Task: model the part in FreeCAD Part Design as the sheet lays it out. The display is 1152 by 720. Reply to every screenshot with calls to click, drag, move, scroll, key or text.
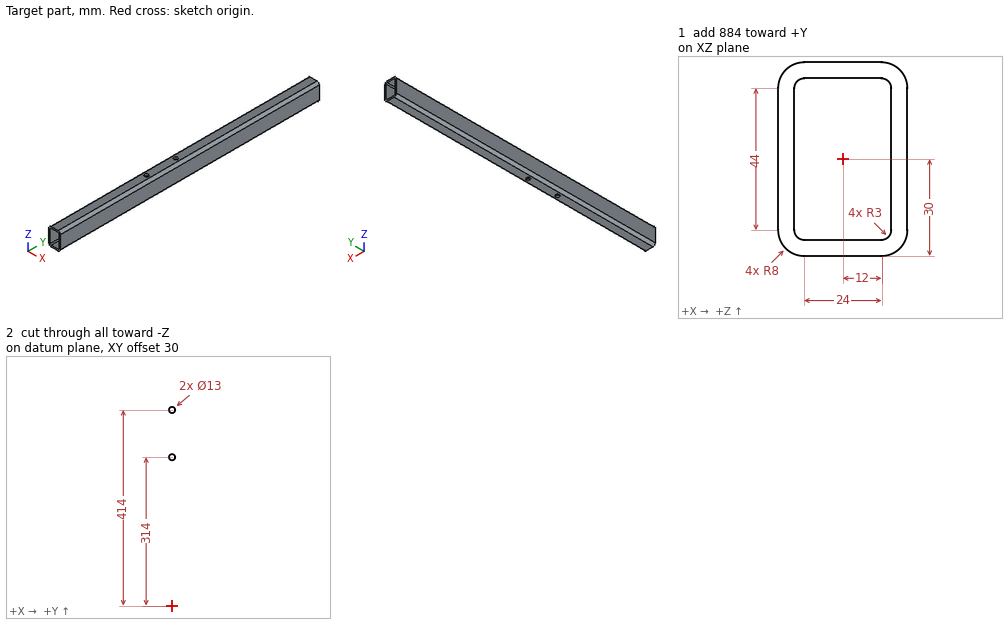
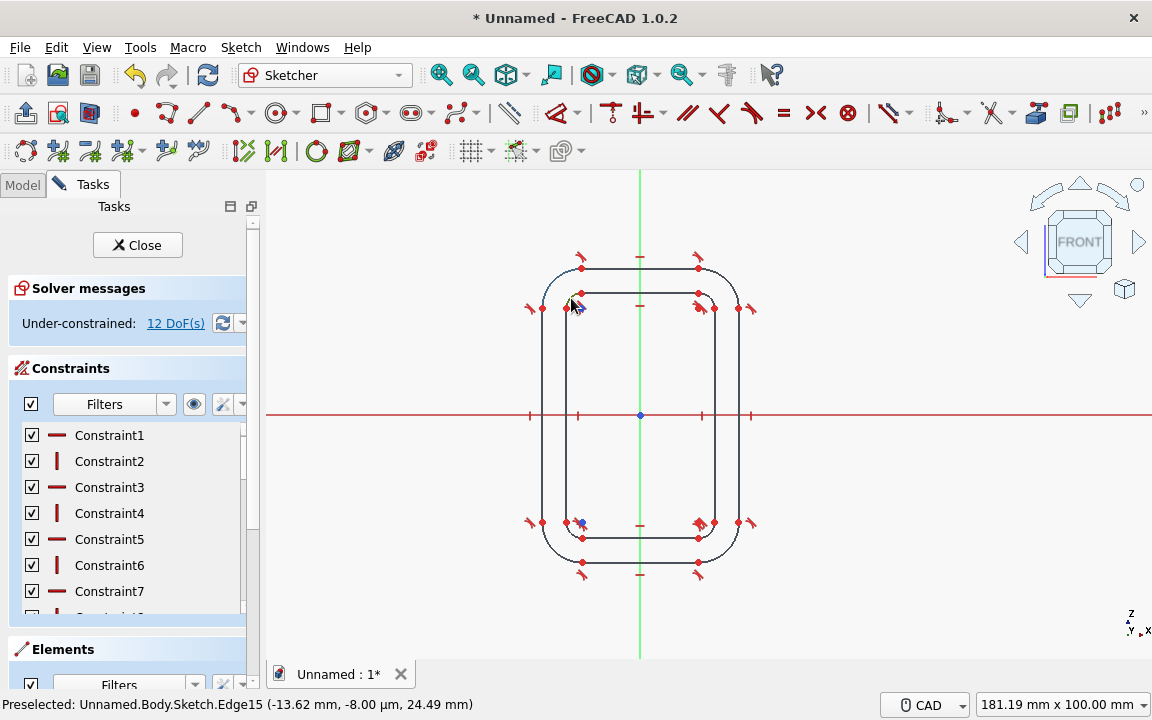
click(612, 114)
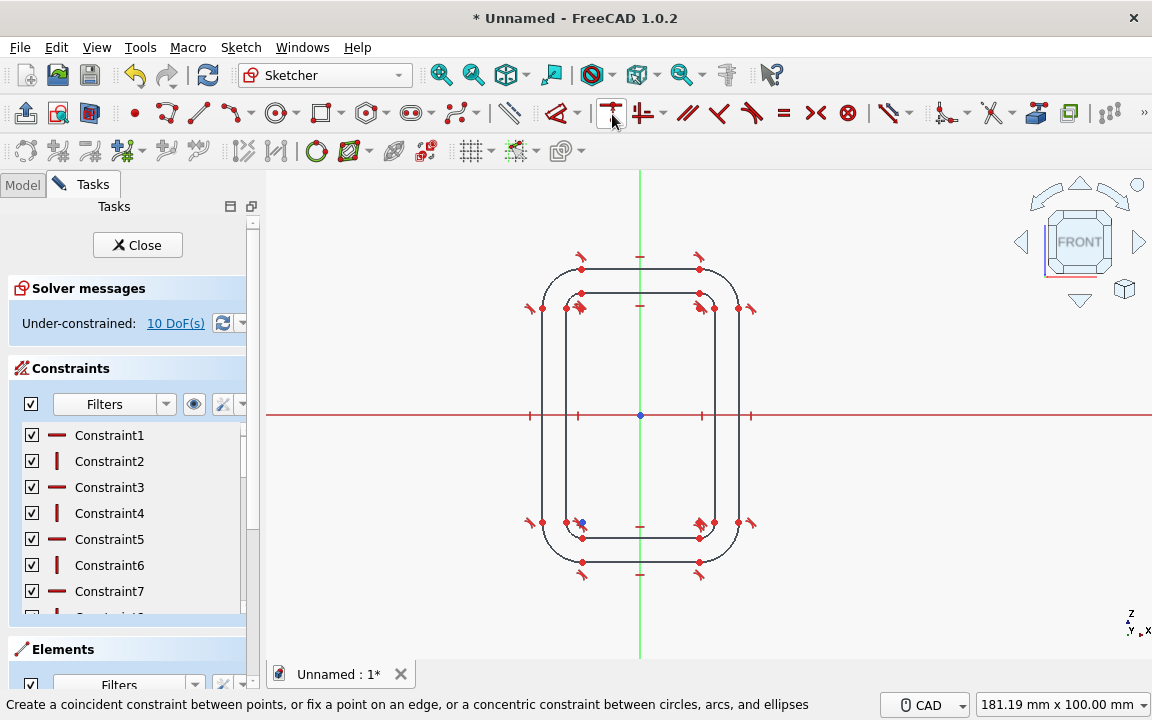
click(547, 541)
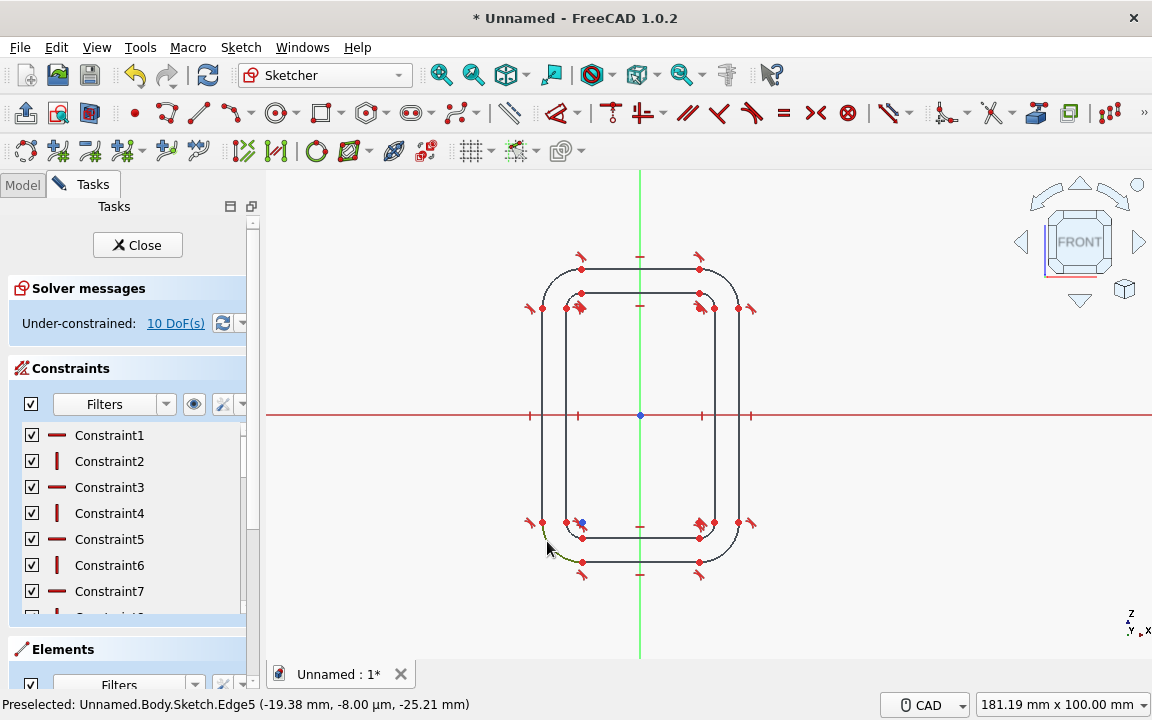
click(564, 273)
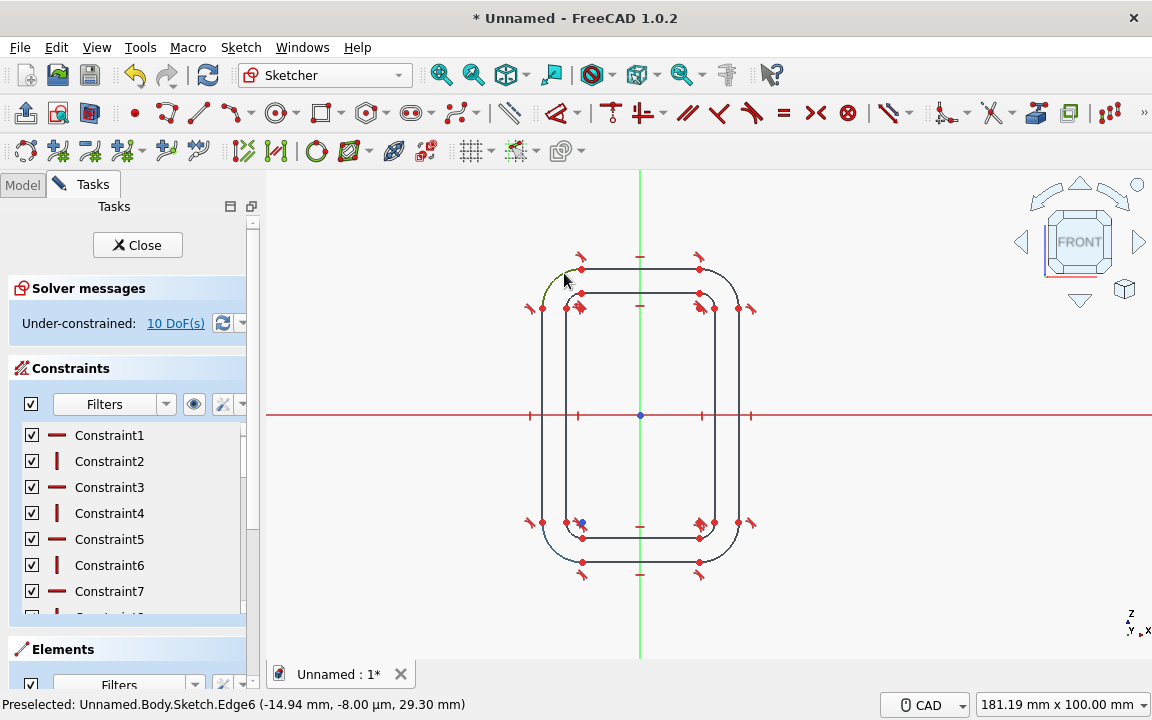
click(735, 291)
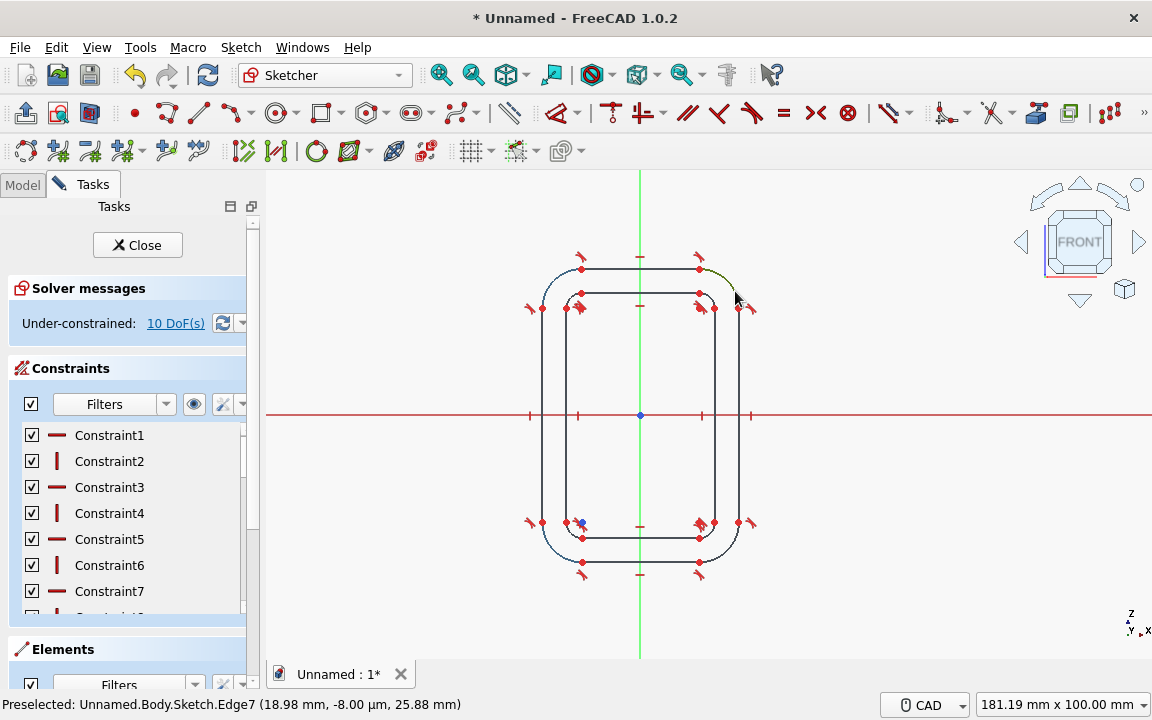
click(717, 558)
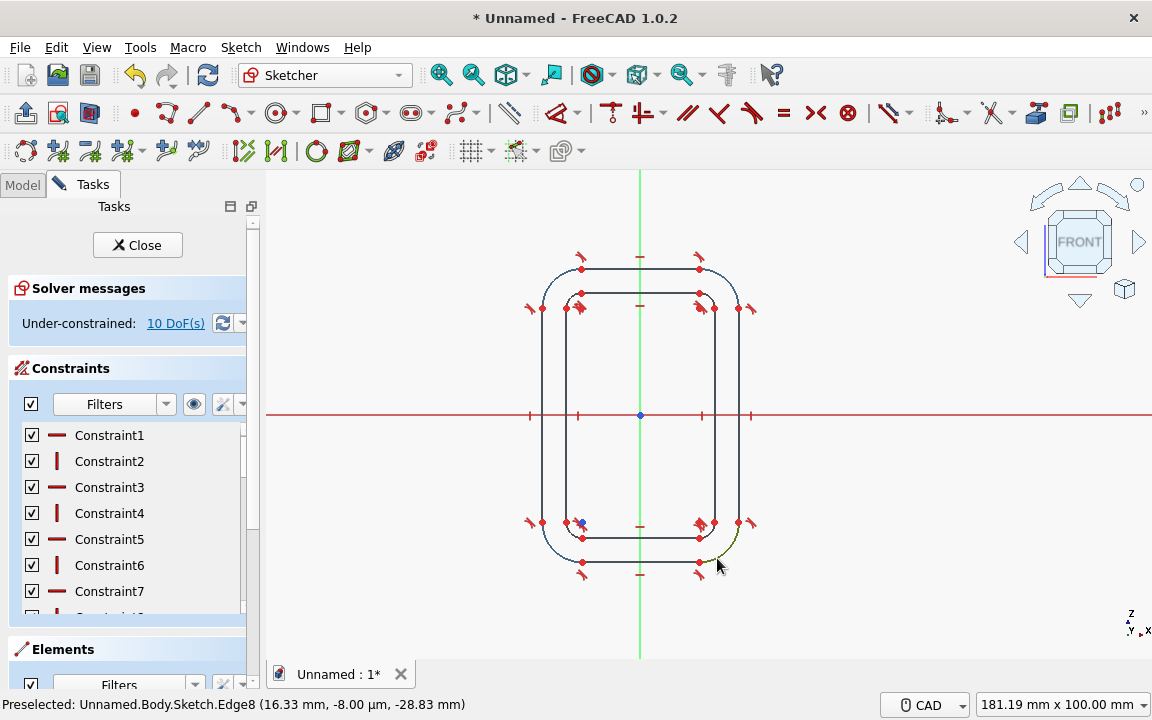
key(e)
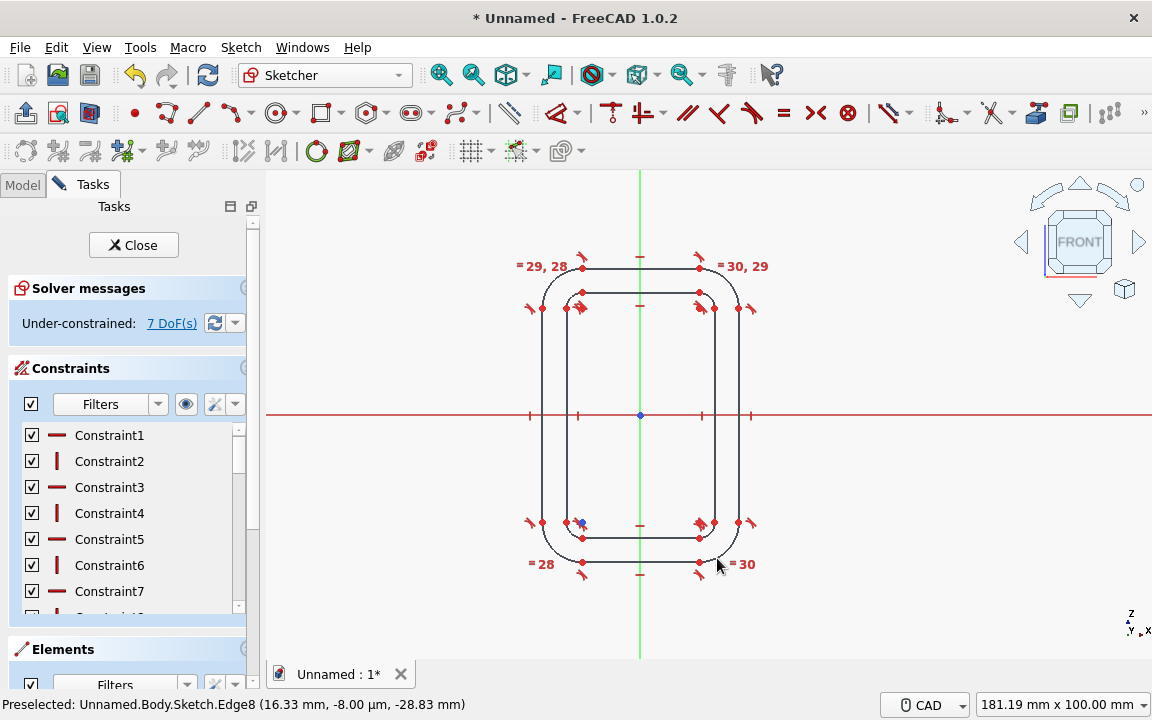
click(710, 533)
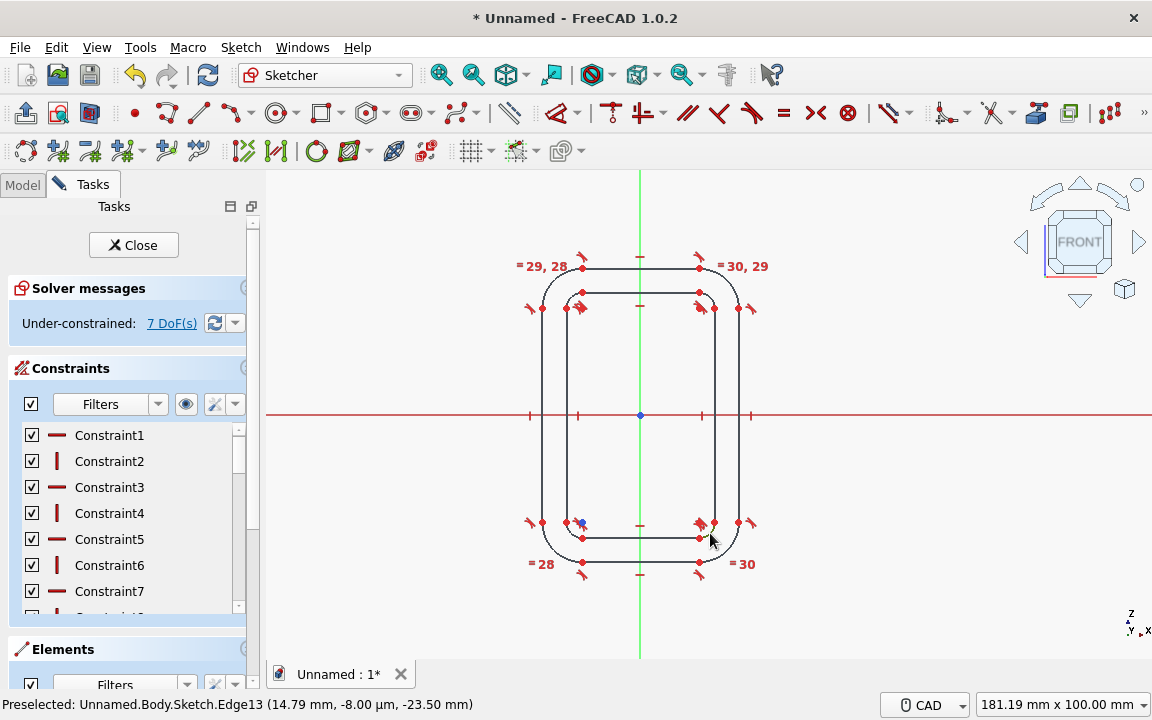
click(571, 533)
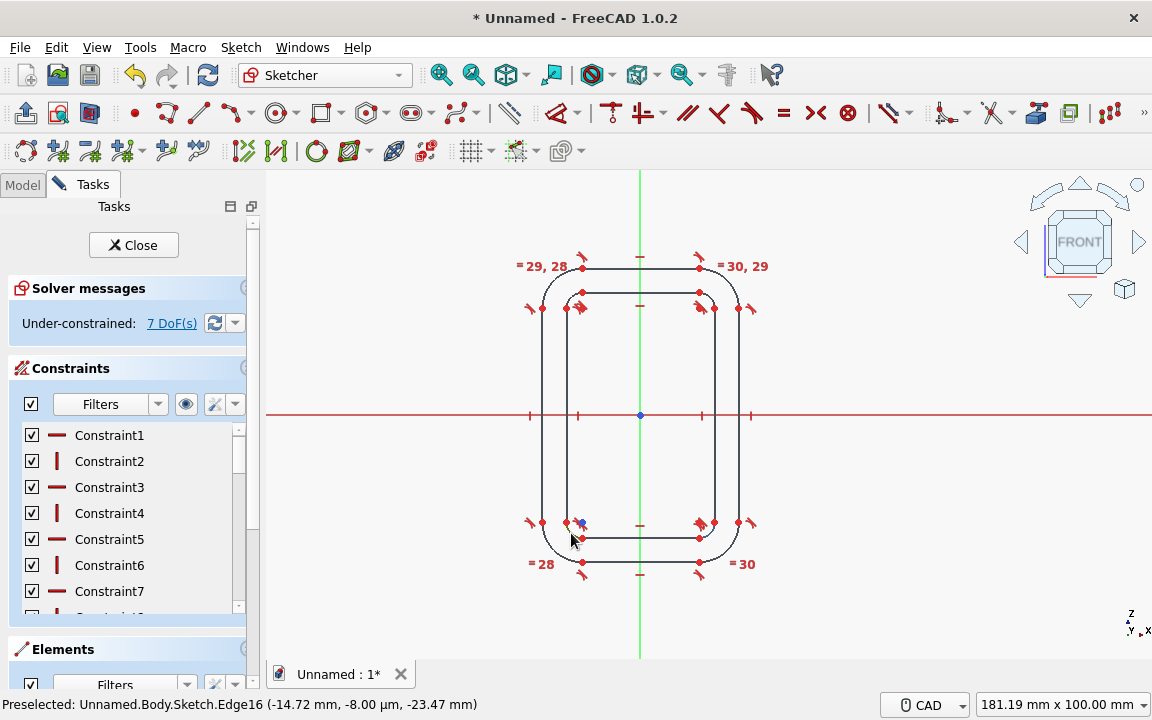
click(784, 114)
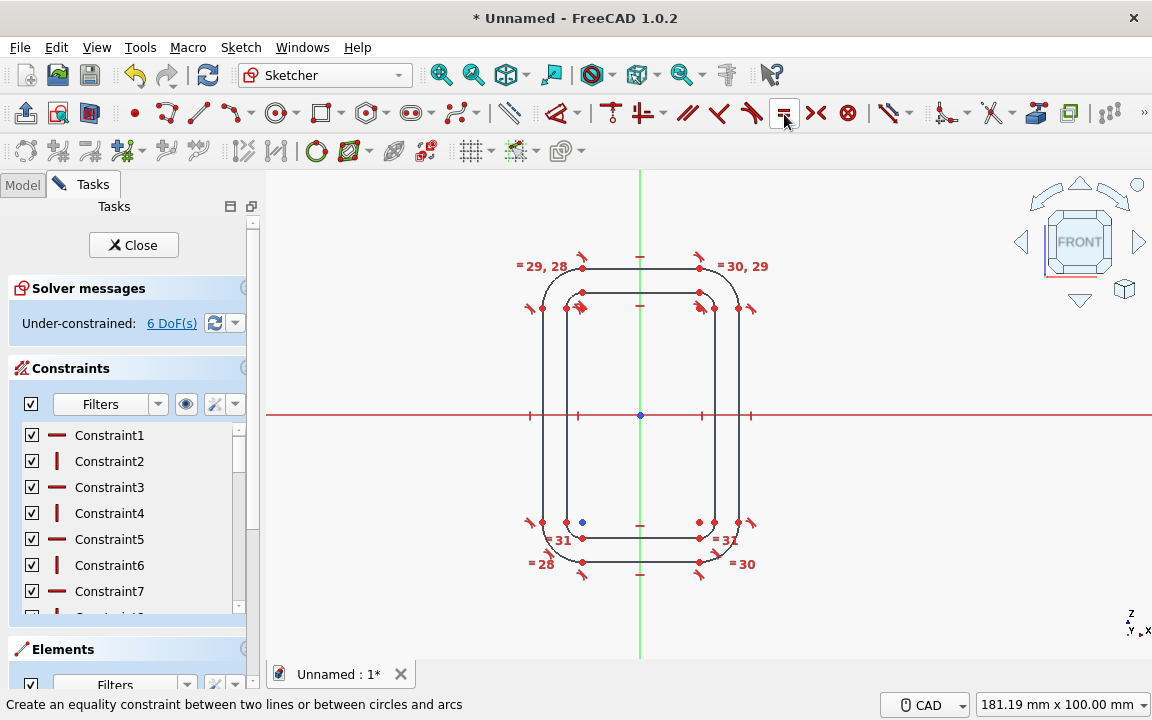
scroll(547, 540, up, 4)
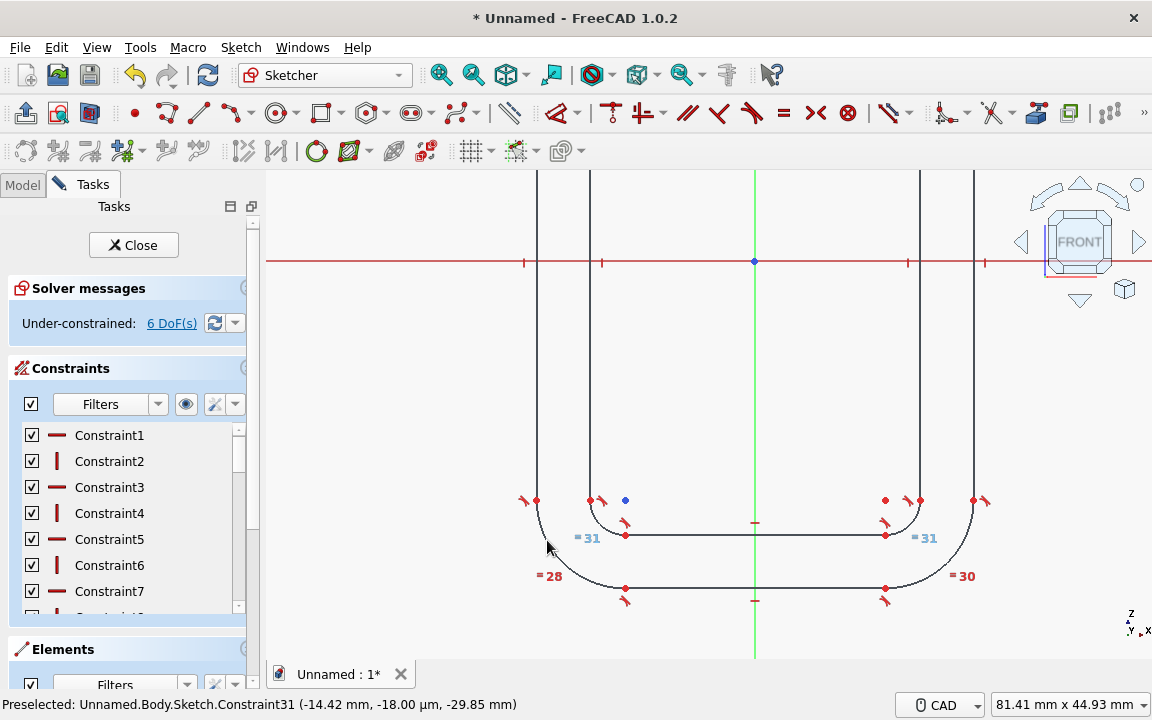
click(546, 540)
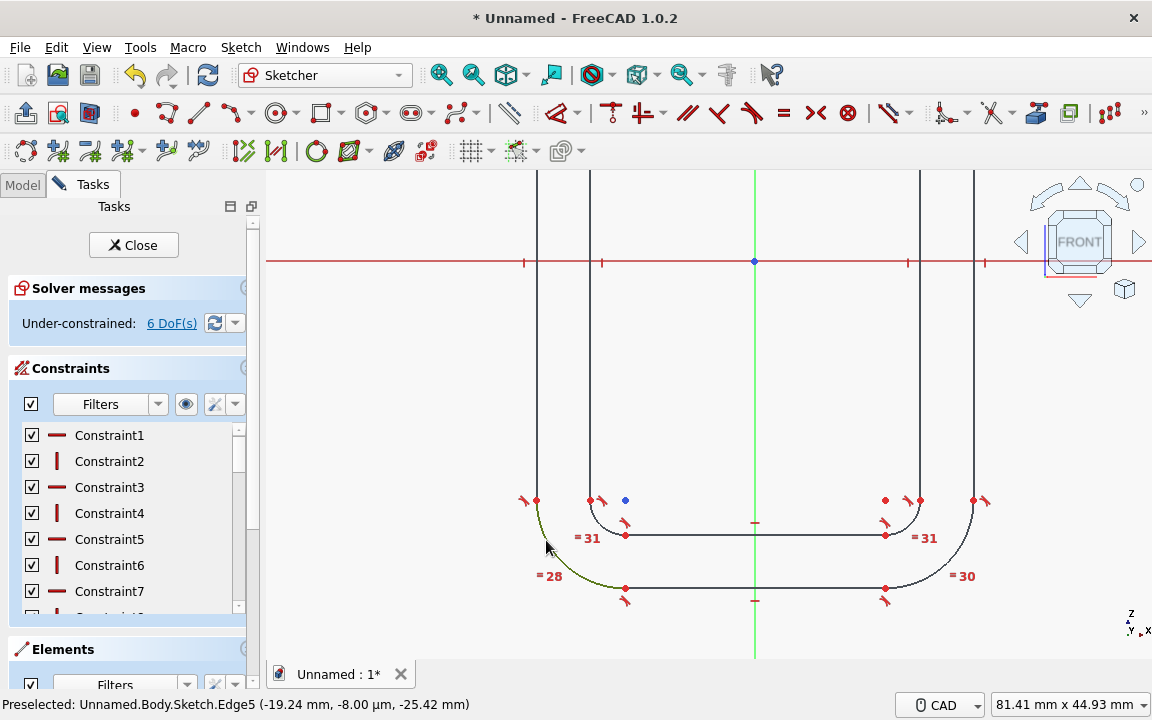
click(580, 114)